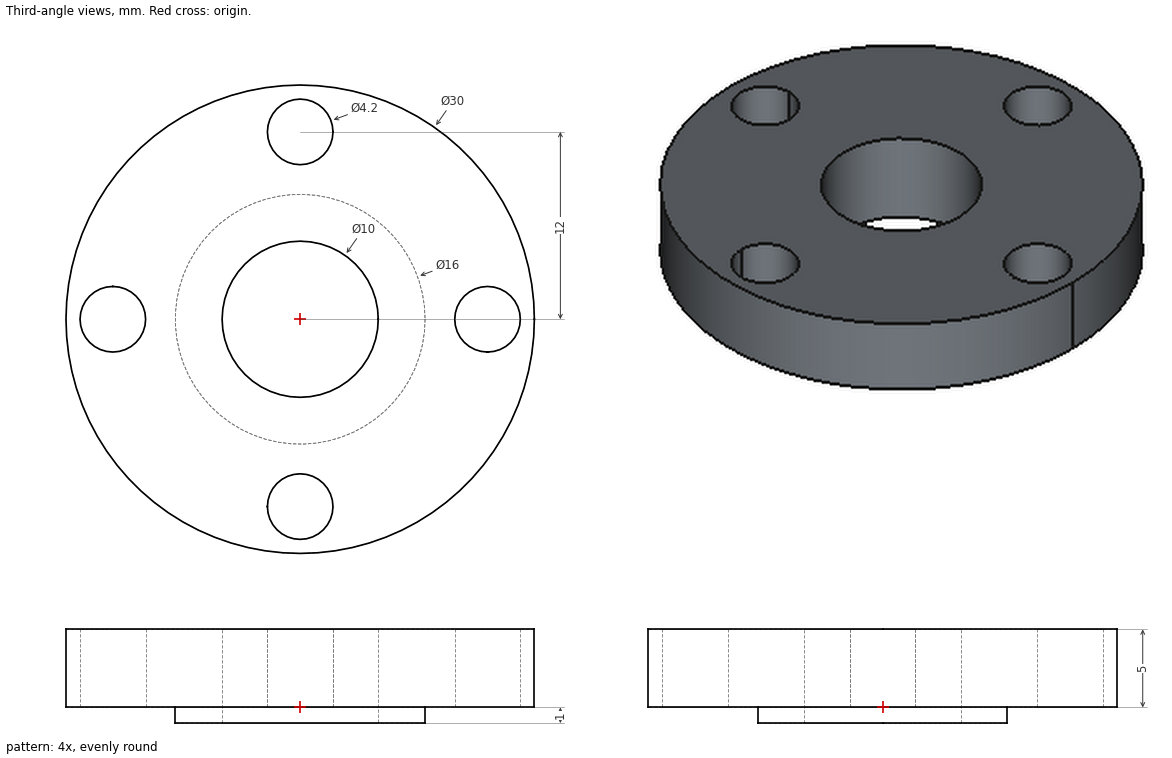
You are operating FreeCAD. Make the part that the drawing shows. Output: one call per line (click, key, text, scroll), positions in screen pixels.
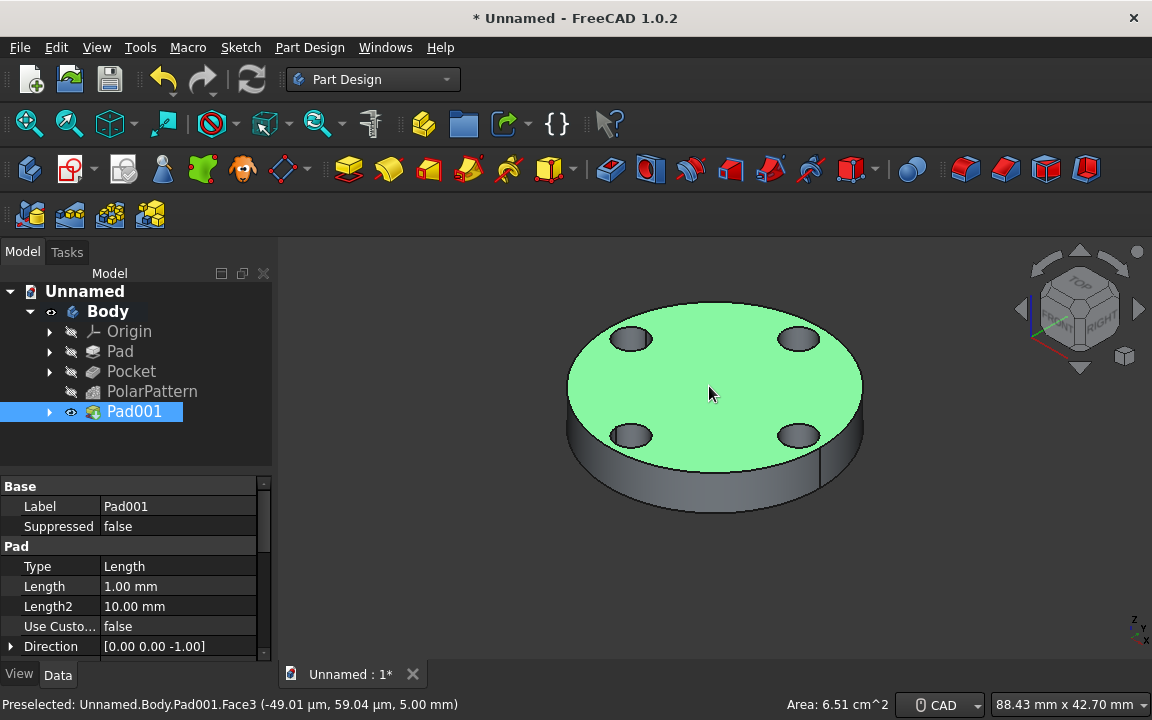
click(70, 170)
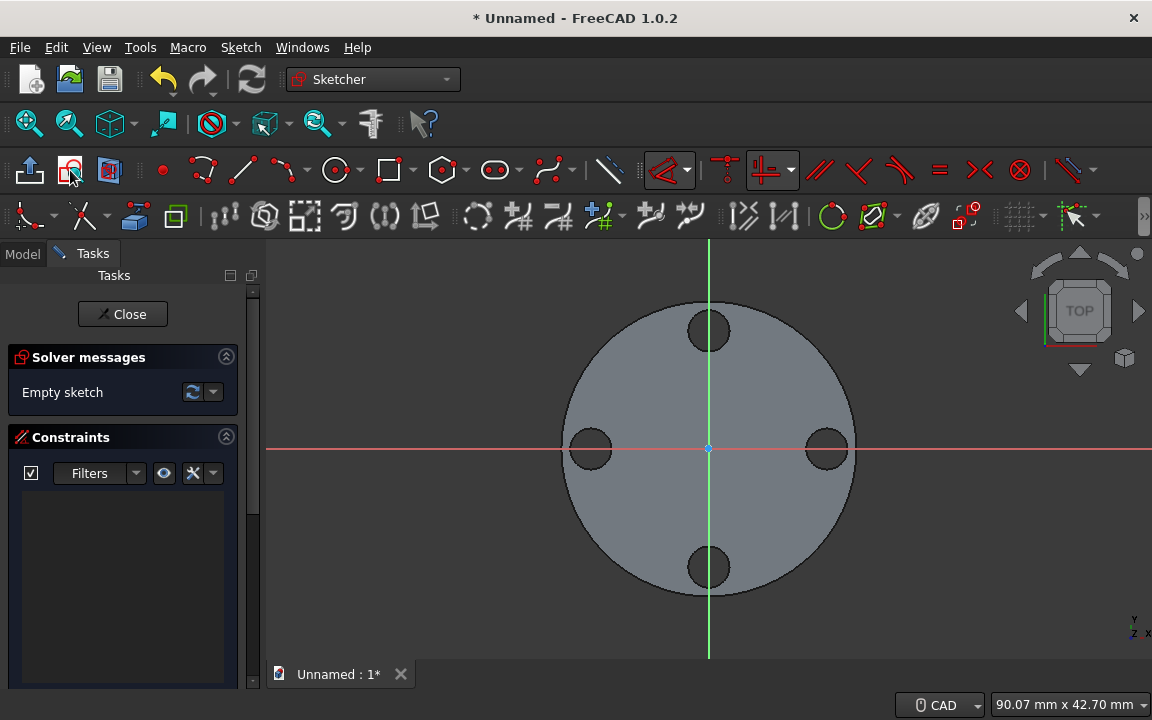
scroll(749, 449, up, 5)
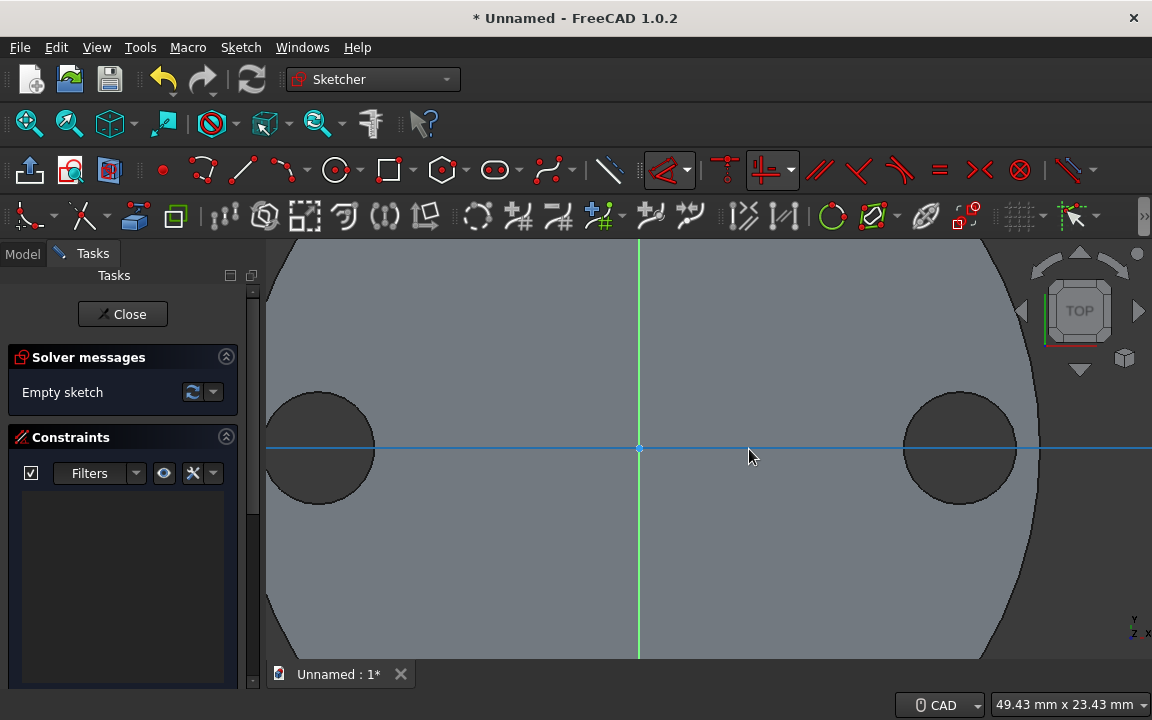
click(336, 170)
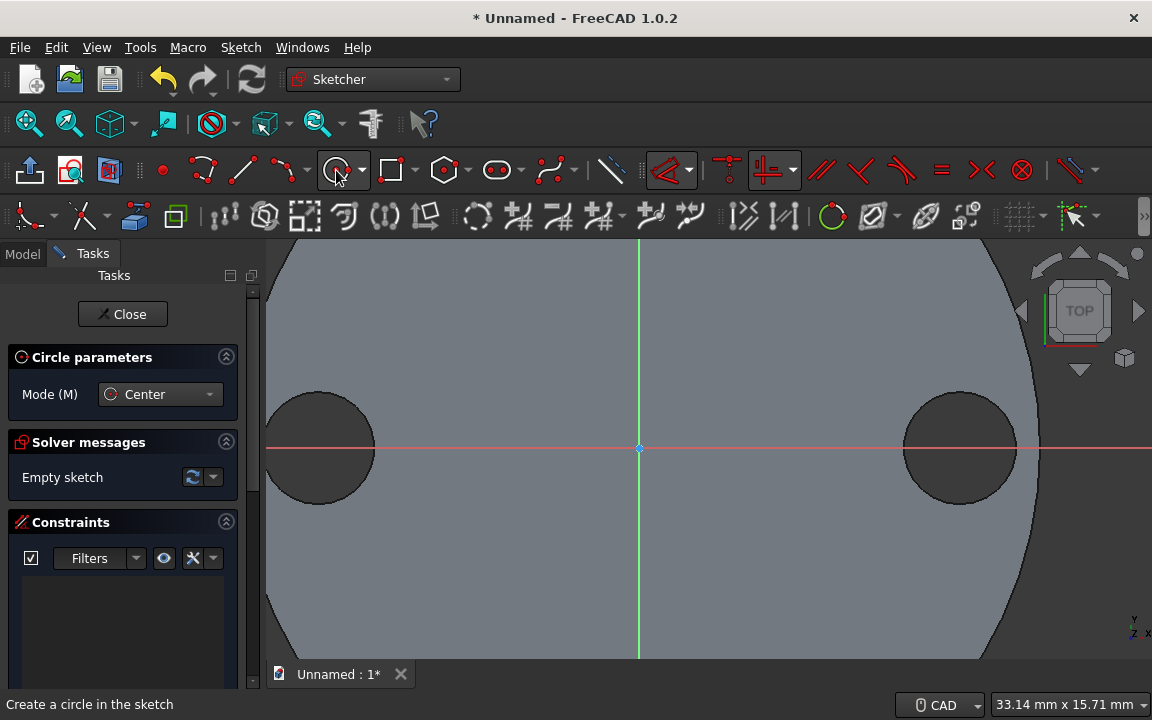
click(639, 448)
click(734, 354)
key(Escape)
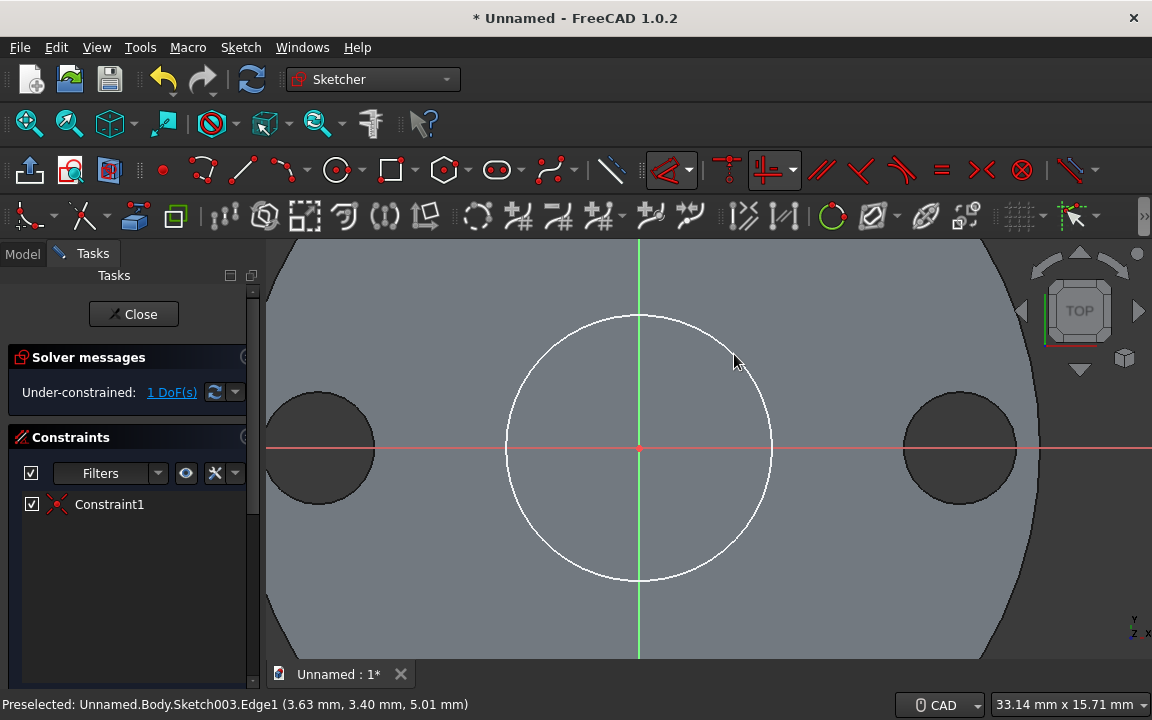
click(733, 354)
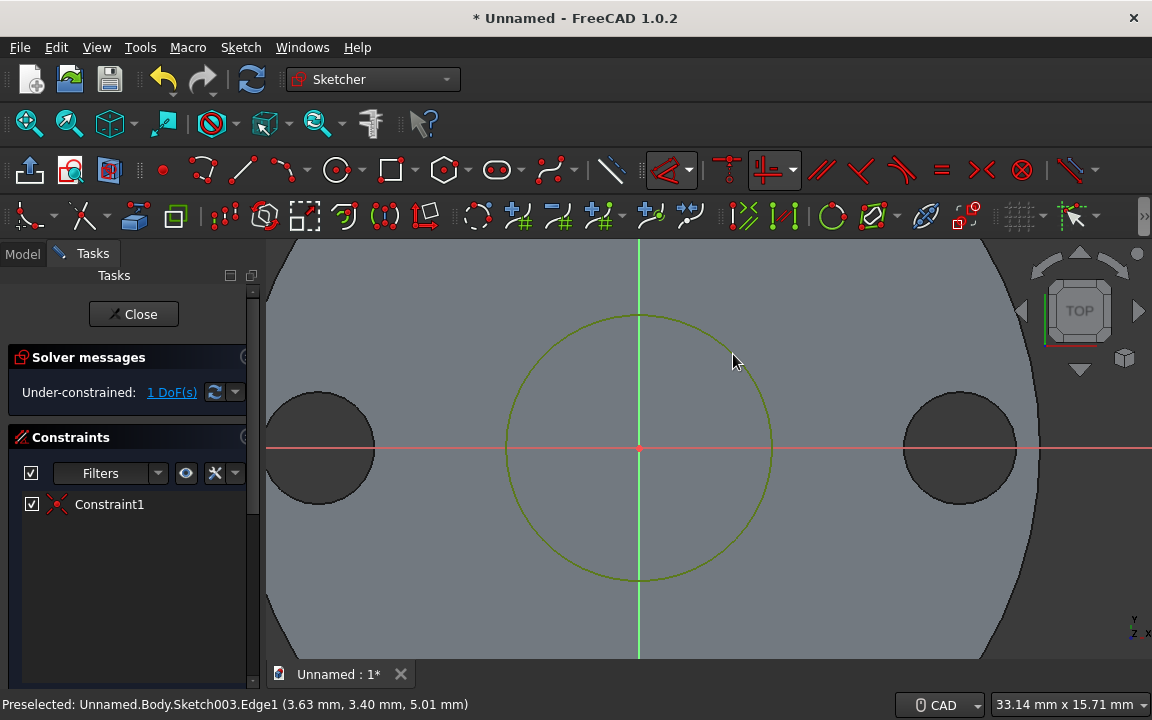
click(692, 170)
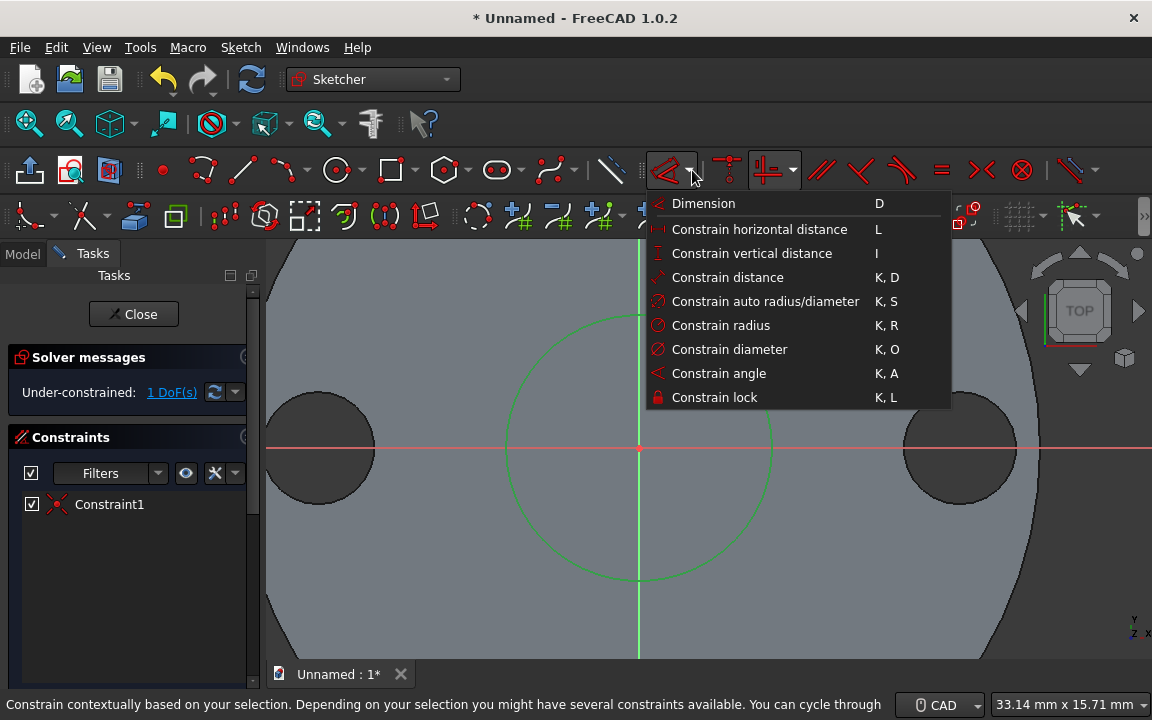
click(799, 349)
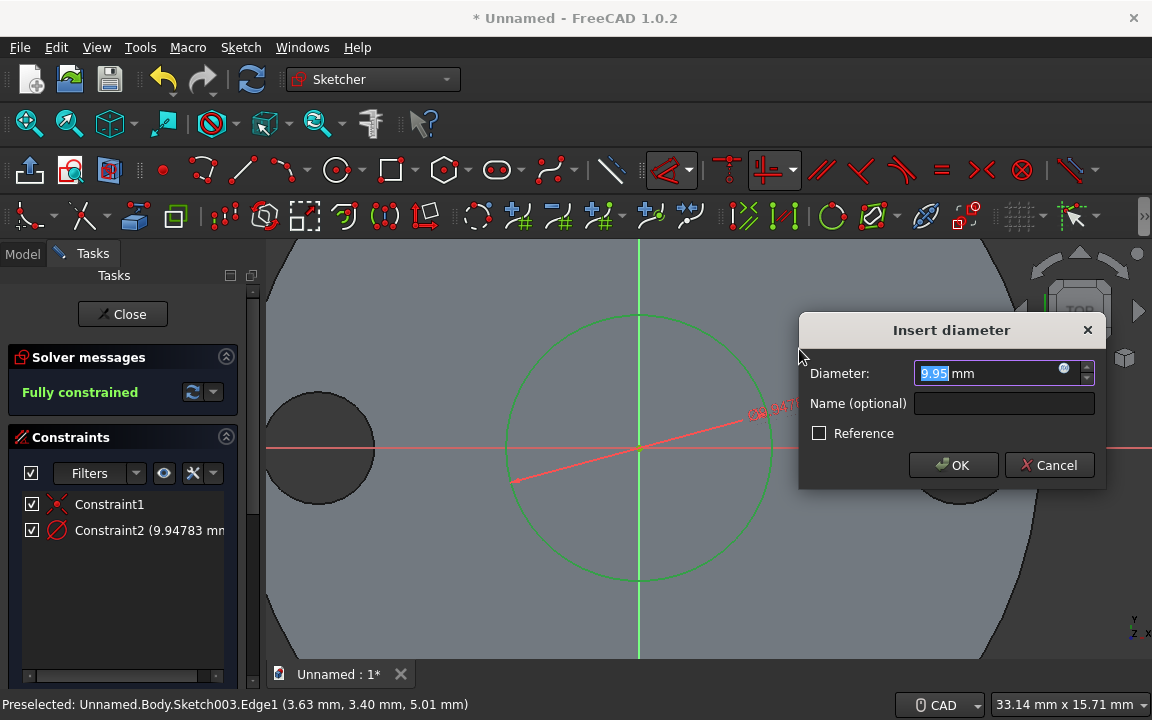
text(10)
key(Return)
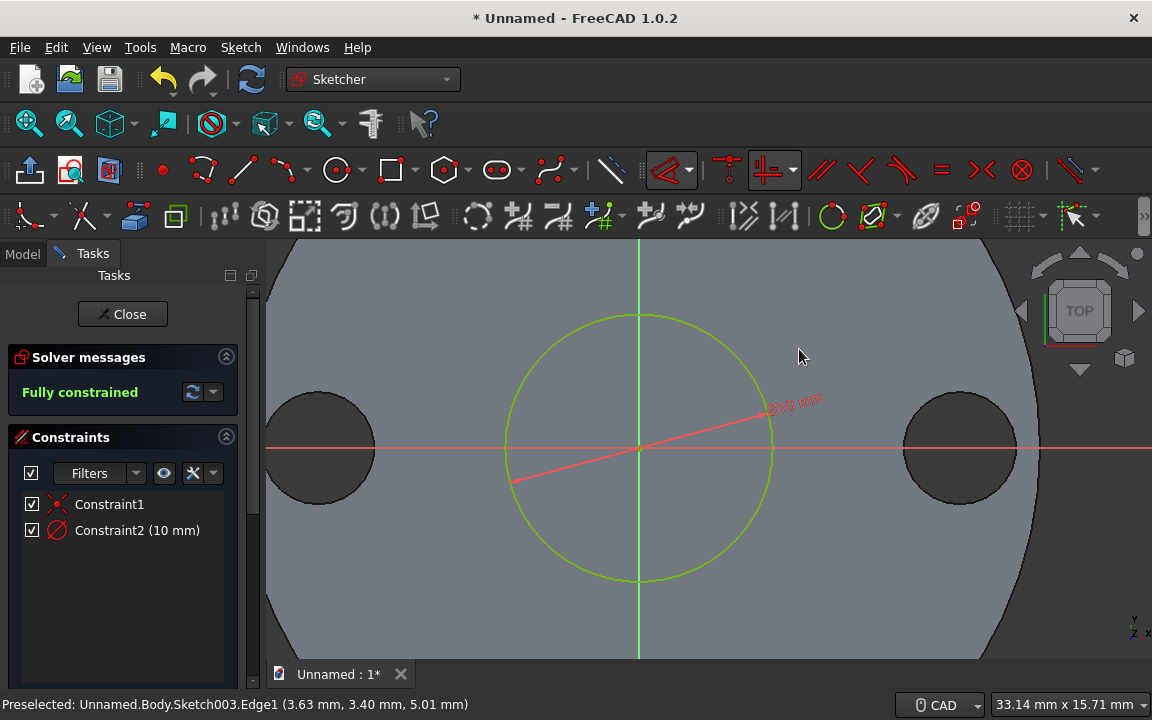
click(123, 314)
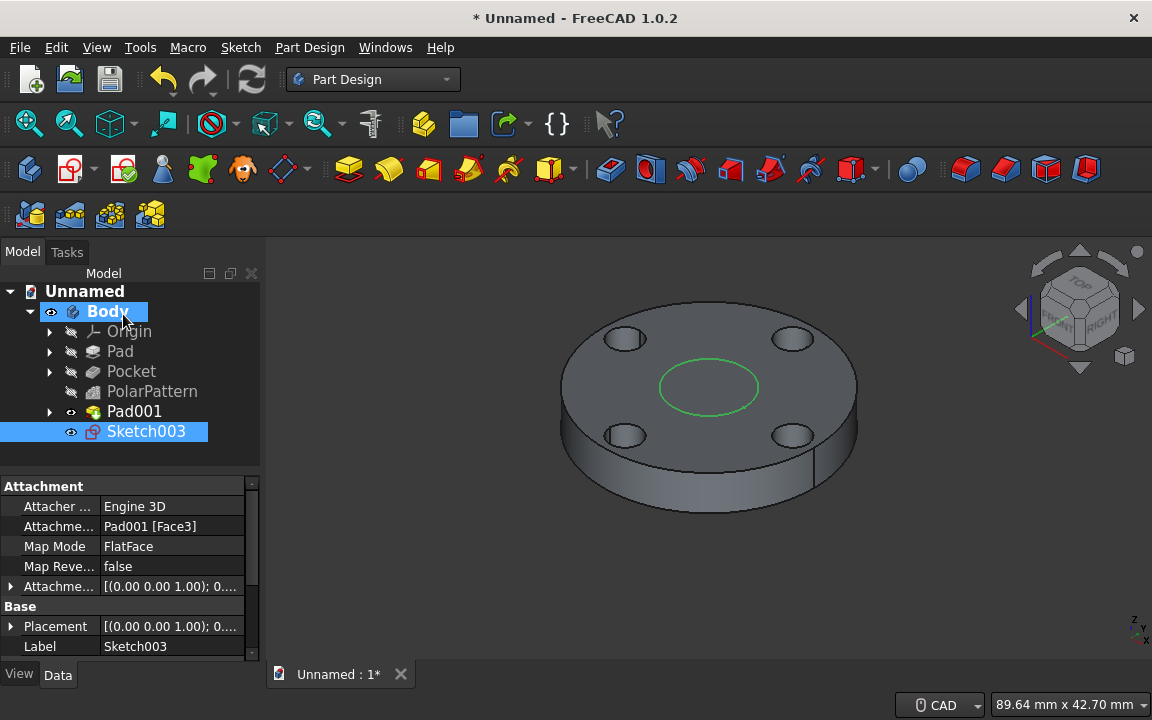
click(612, 170)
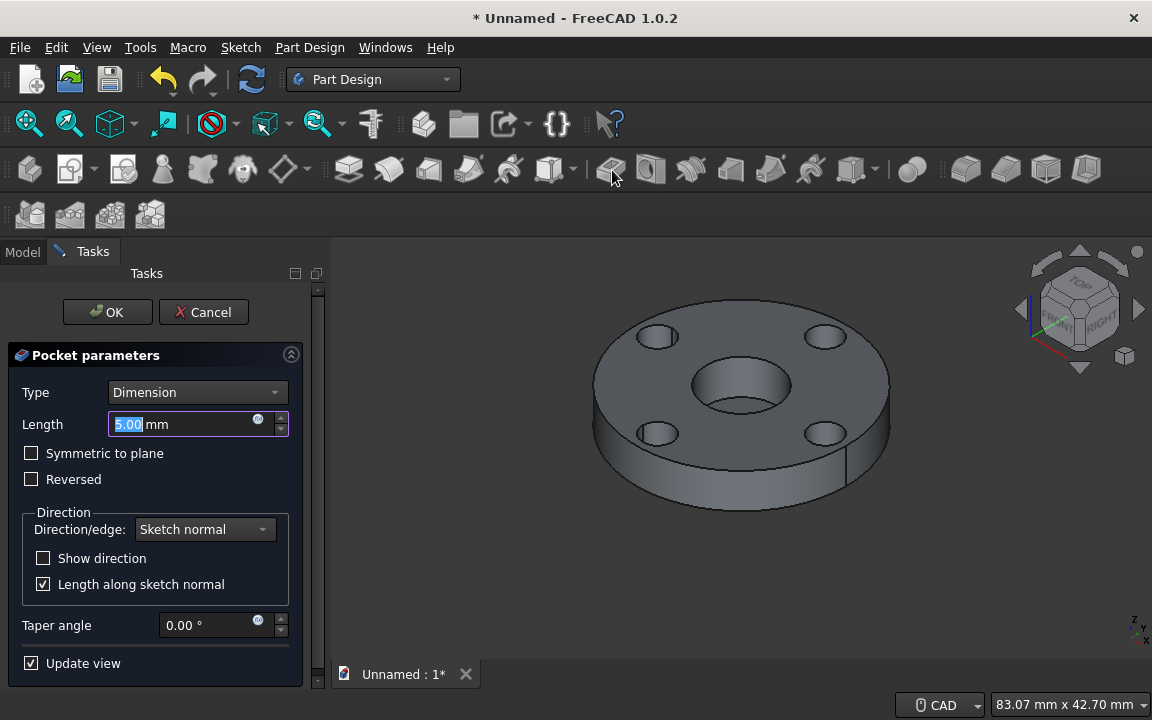
click(198, 392)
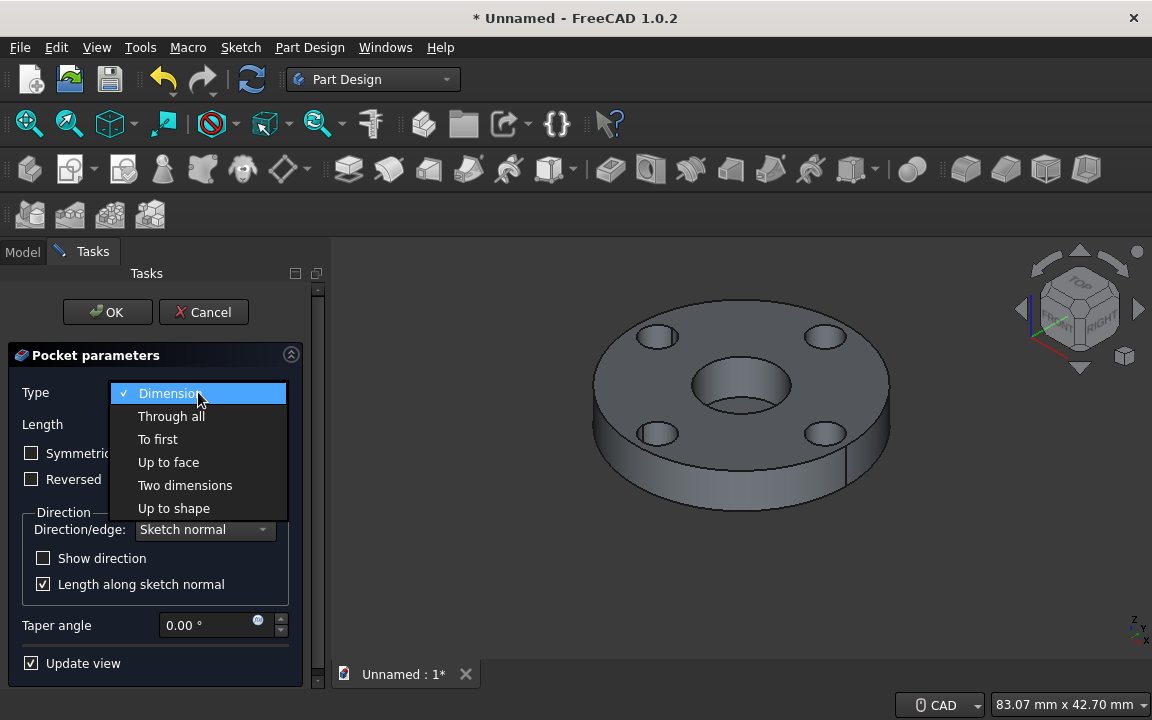
click(198, 416)